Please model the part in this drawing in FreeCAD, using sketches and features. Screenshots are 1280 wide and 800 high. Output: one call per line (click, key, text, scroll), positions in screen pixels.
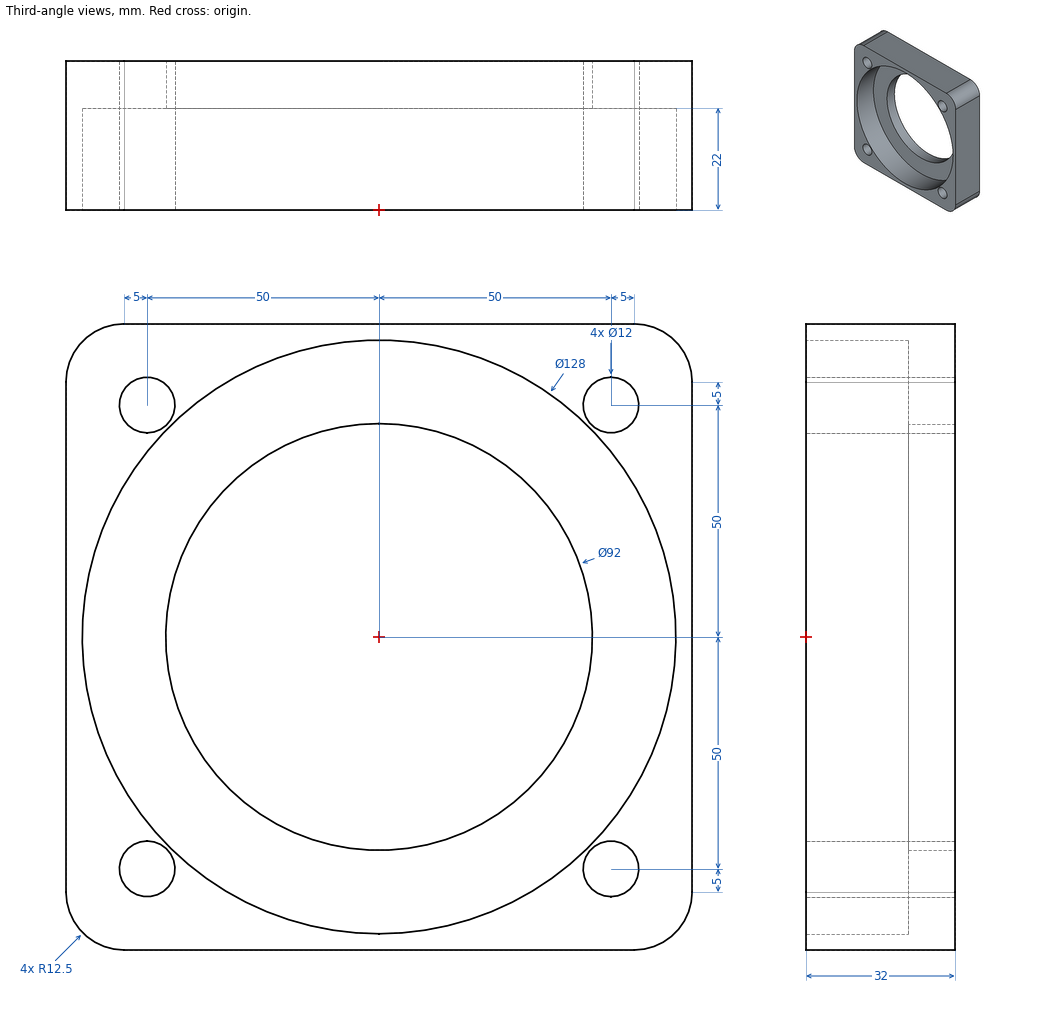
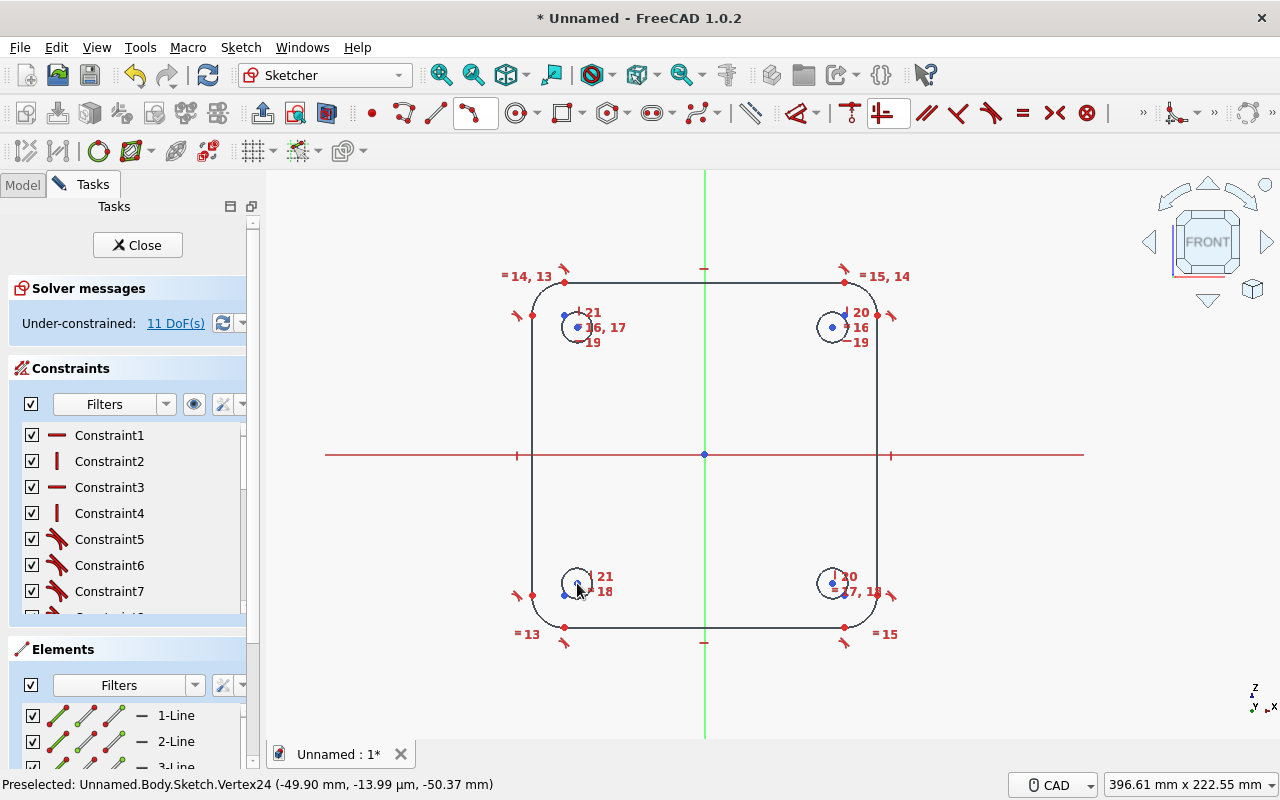
scroll(833, 583, up, 4)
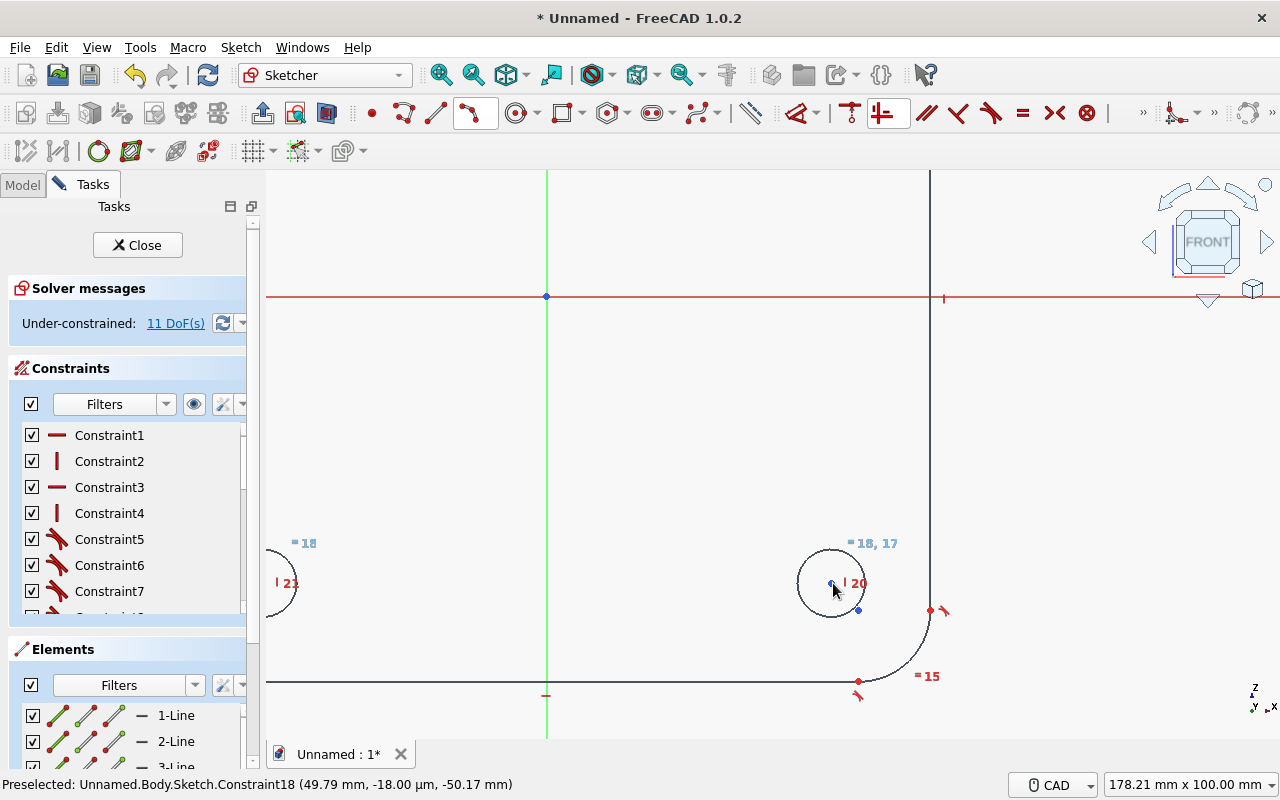
click(831, 583)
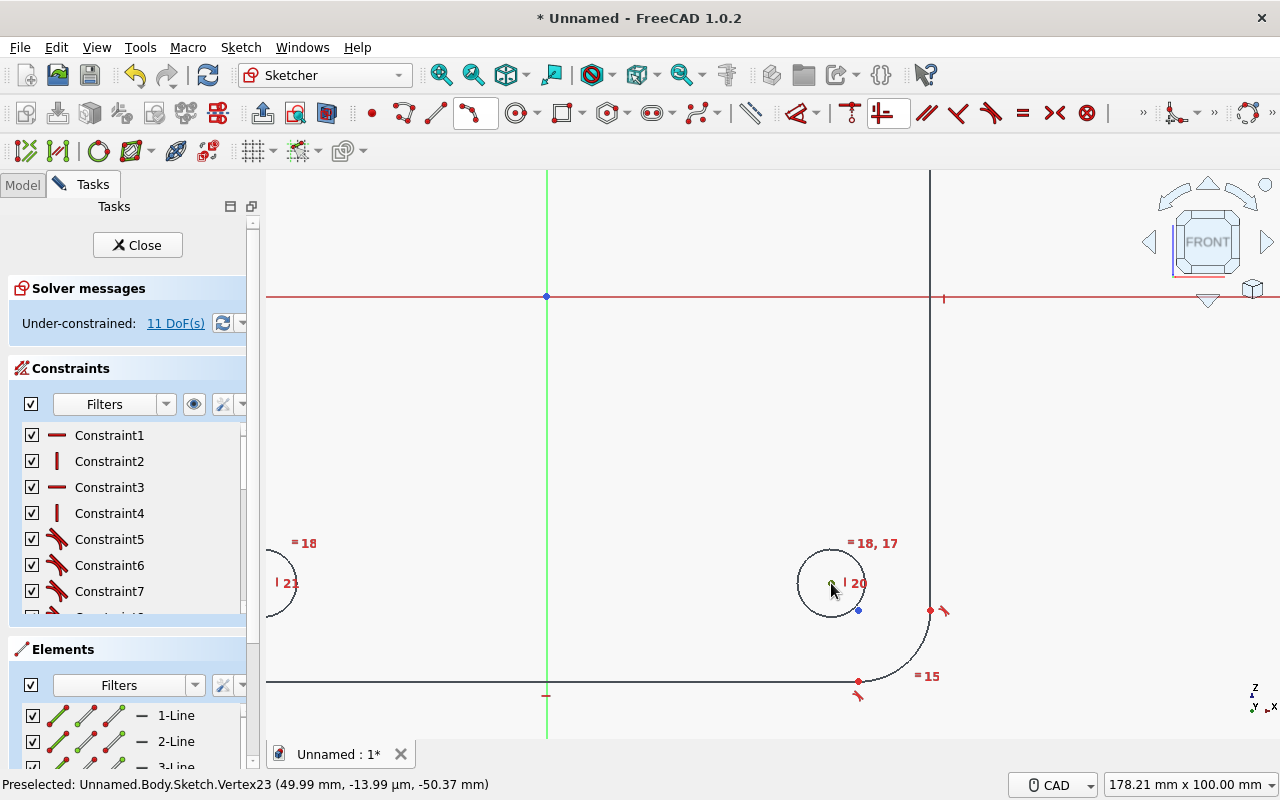
scroll(833, 583, down, 4)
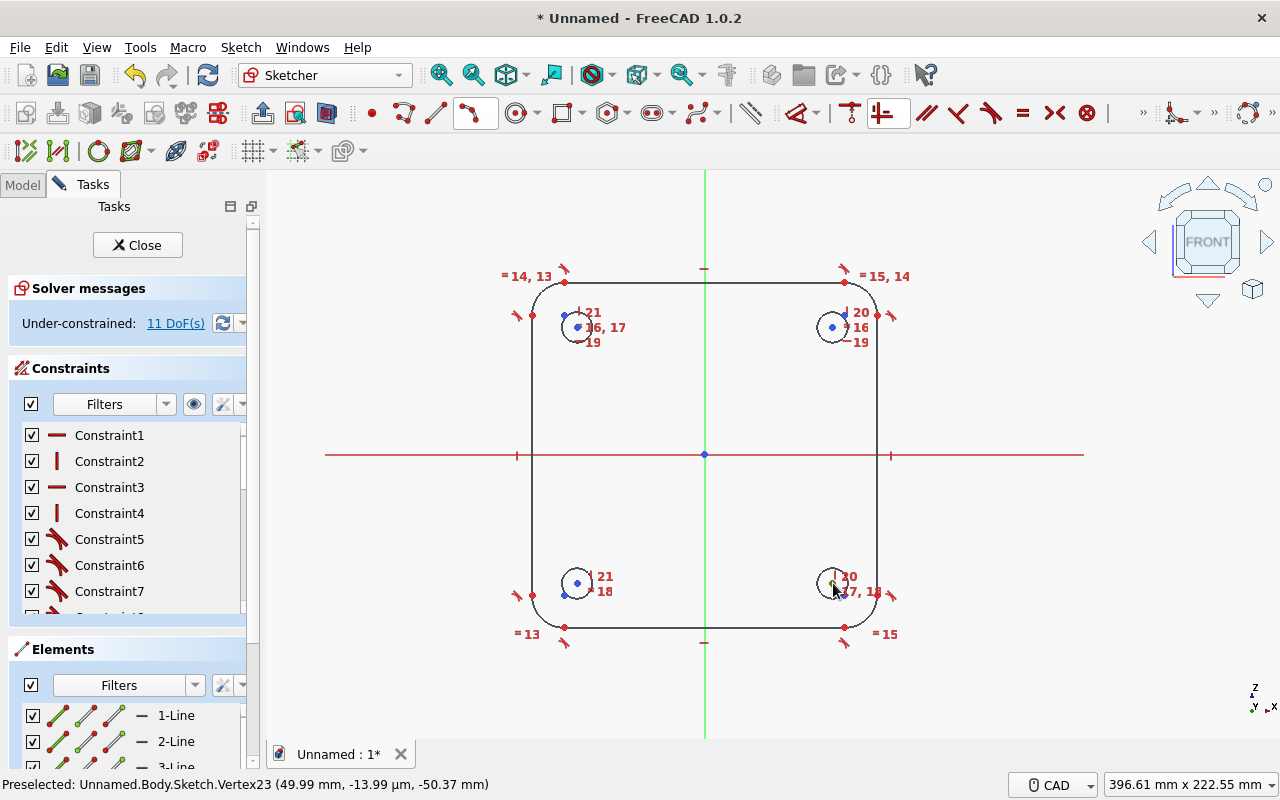
click(577, 583)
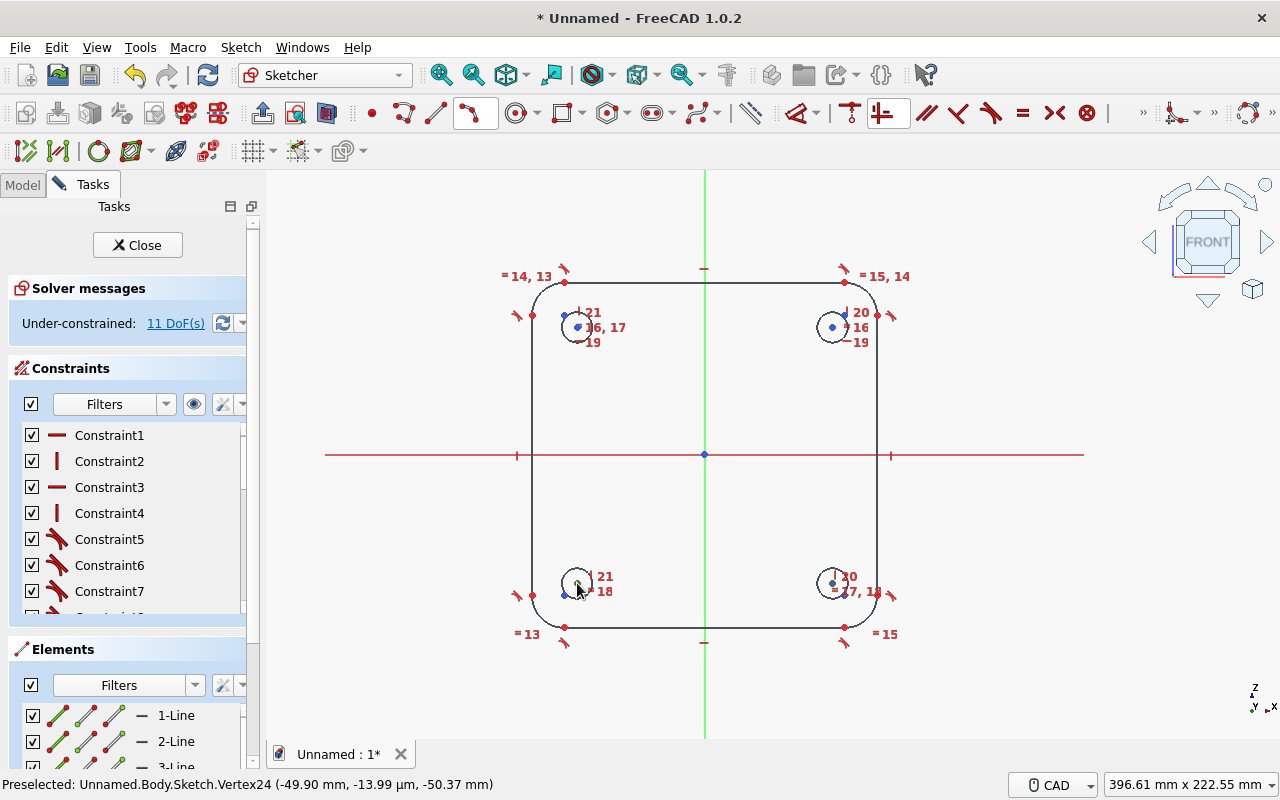
click(904, 114)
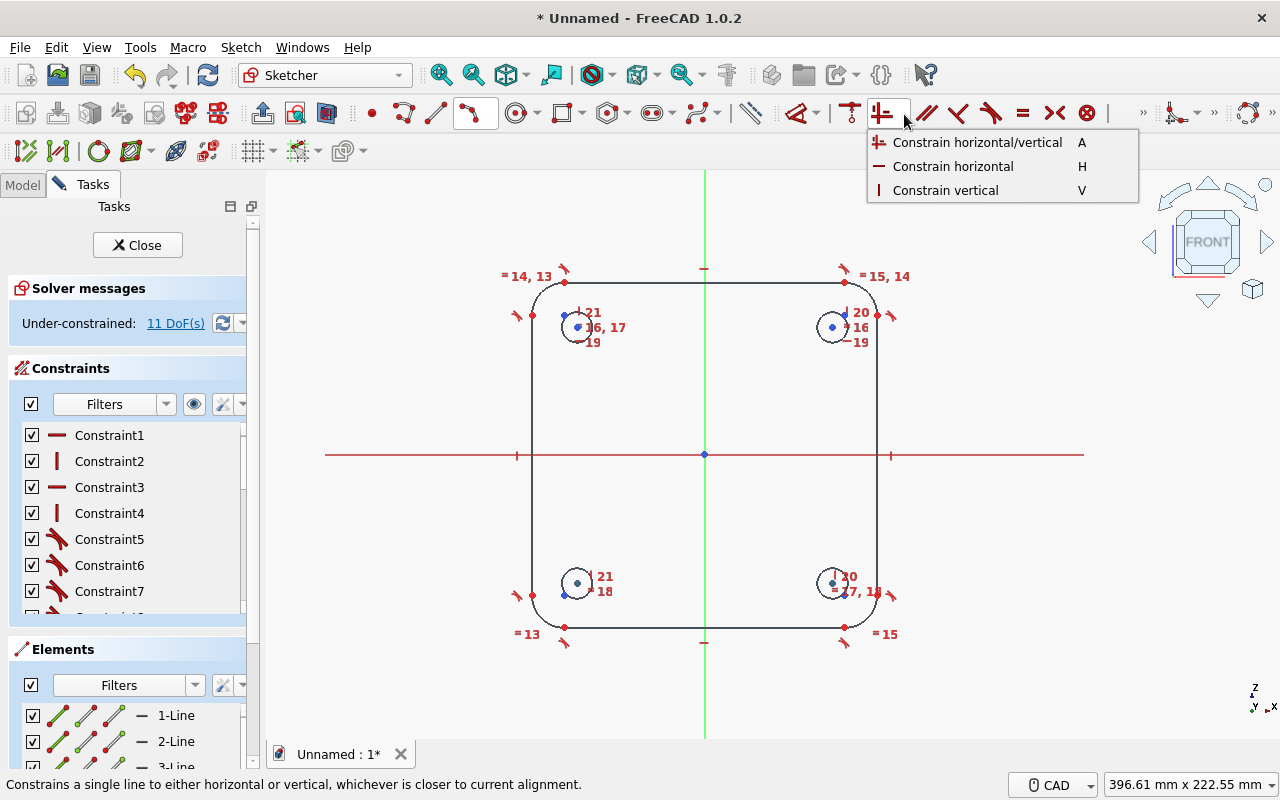
click(1003, 166)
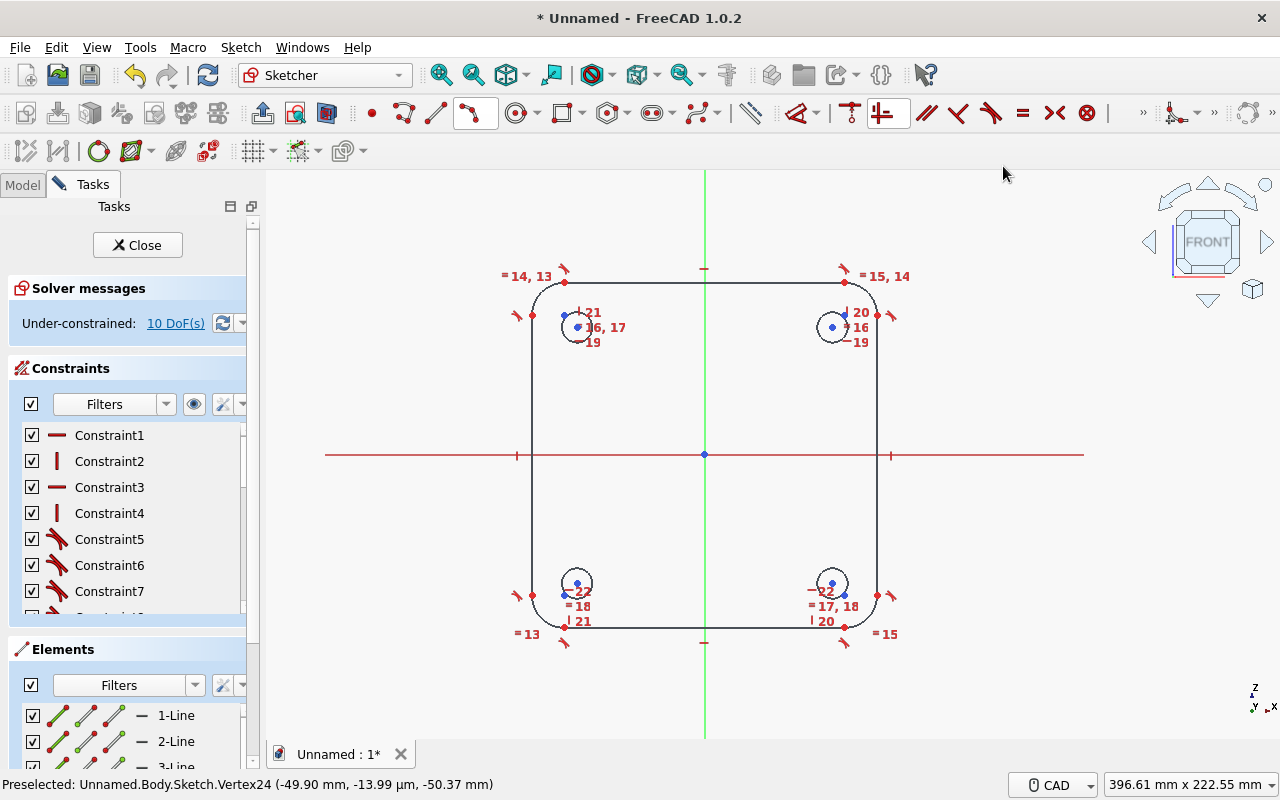
key(d)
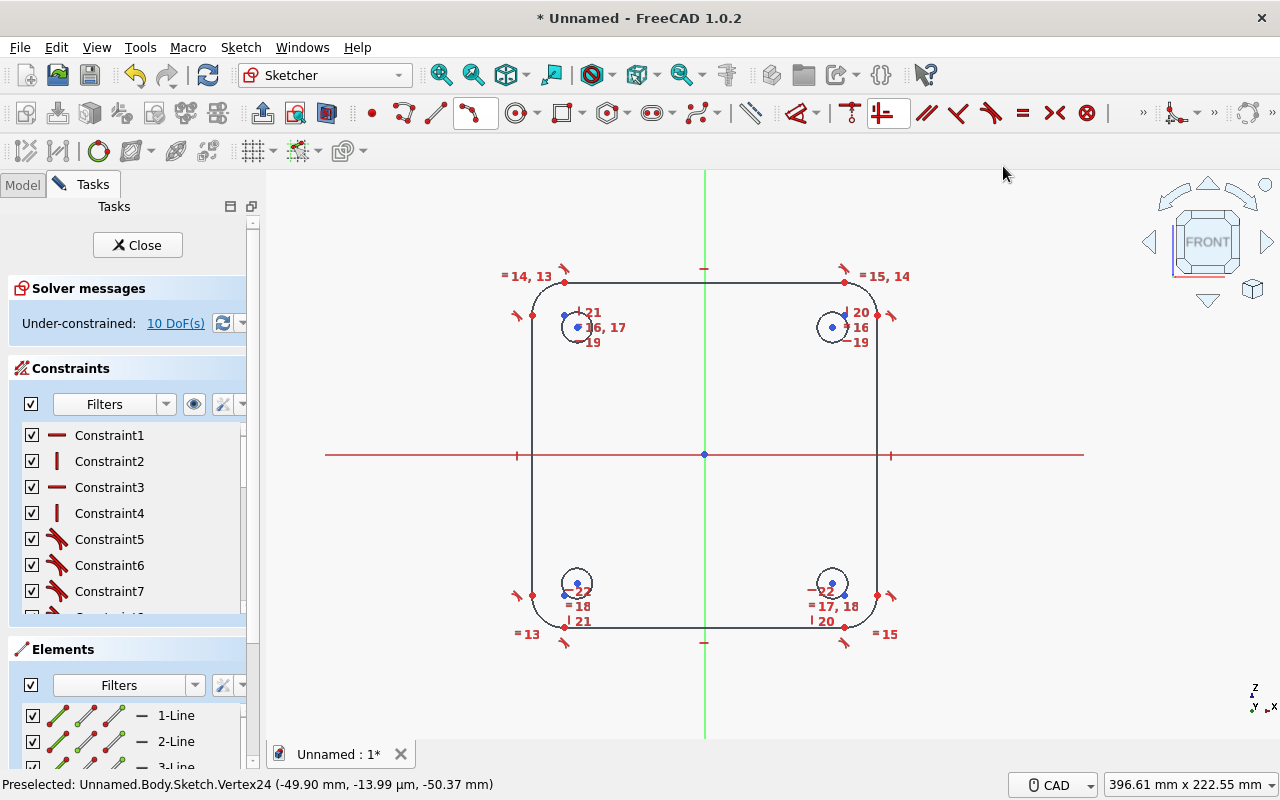
scroll(536, 610, up, 2)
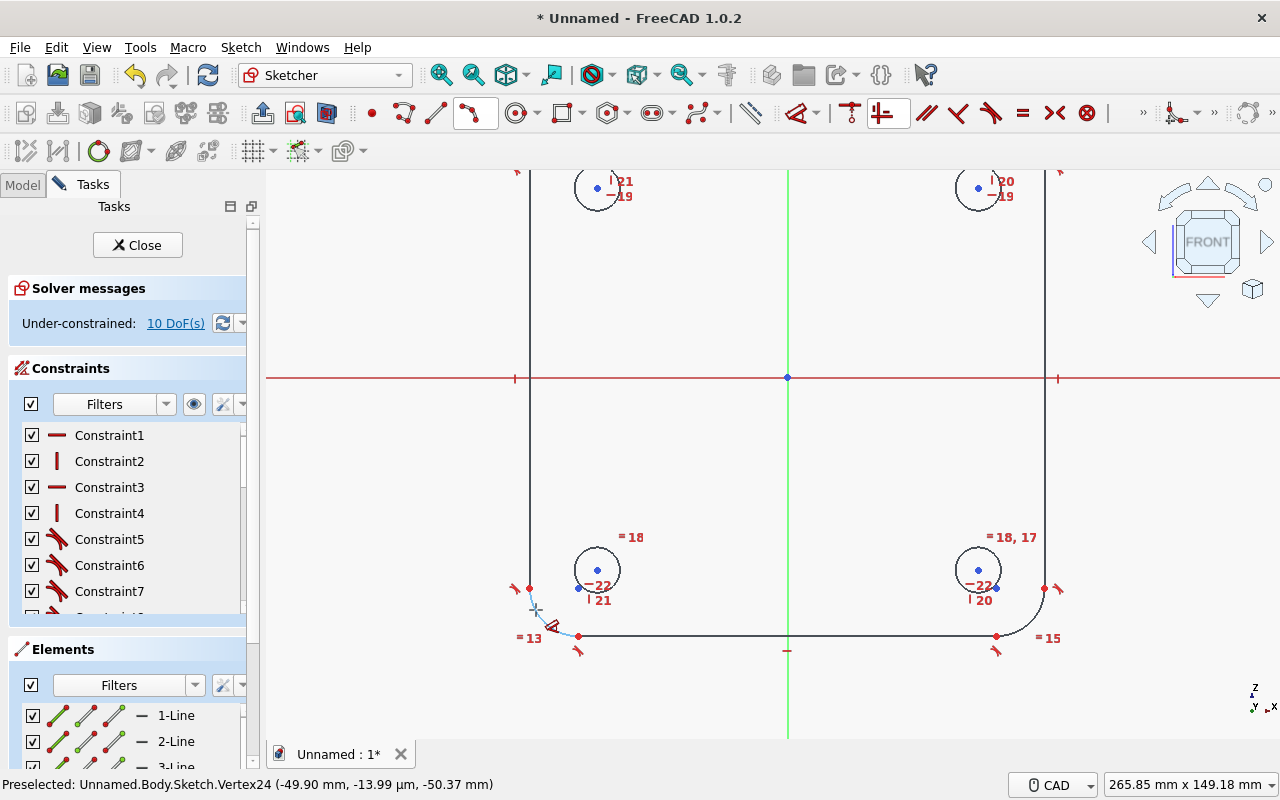
click(535, 610)
click(506, 625)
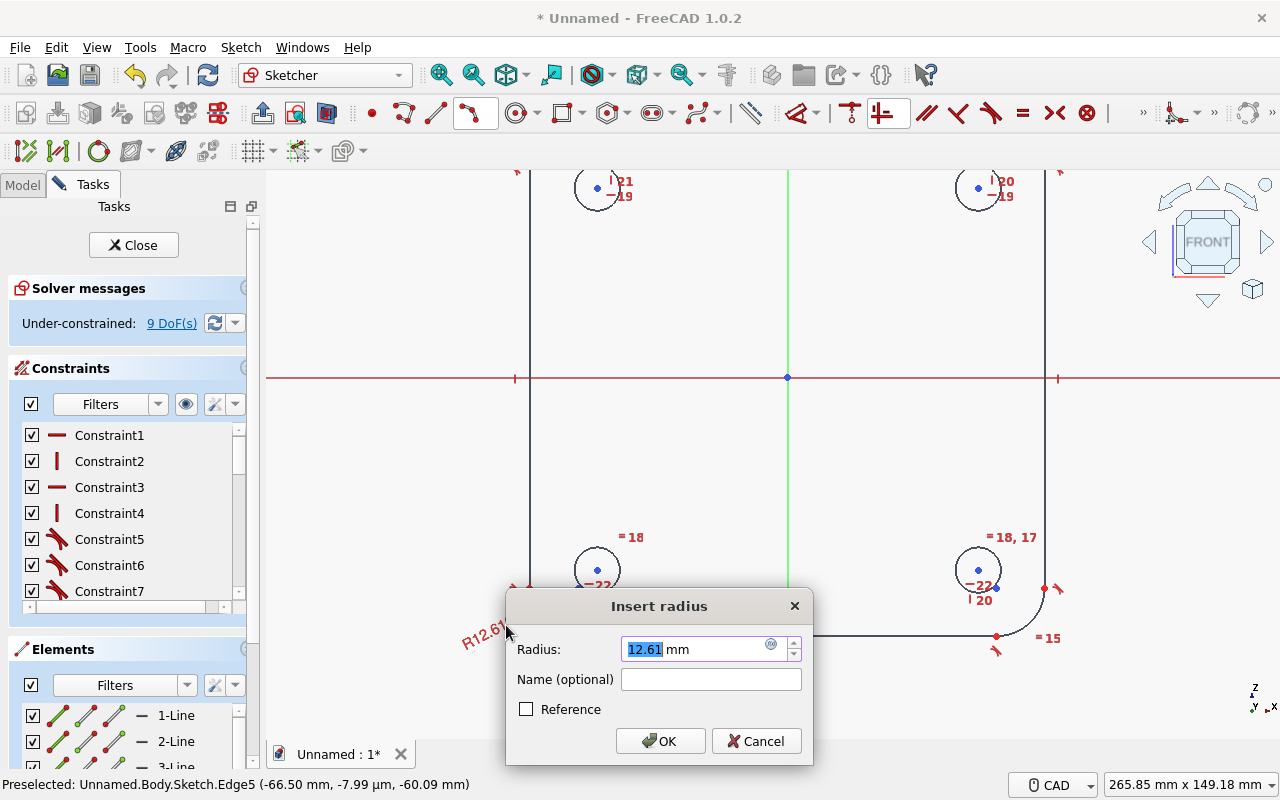
text(12.5)
key(Return)